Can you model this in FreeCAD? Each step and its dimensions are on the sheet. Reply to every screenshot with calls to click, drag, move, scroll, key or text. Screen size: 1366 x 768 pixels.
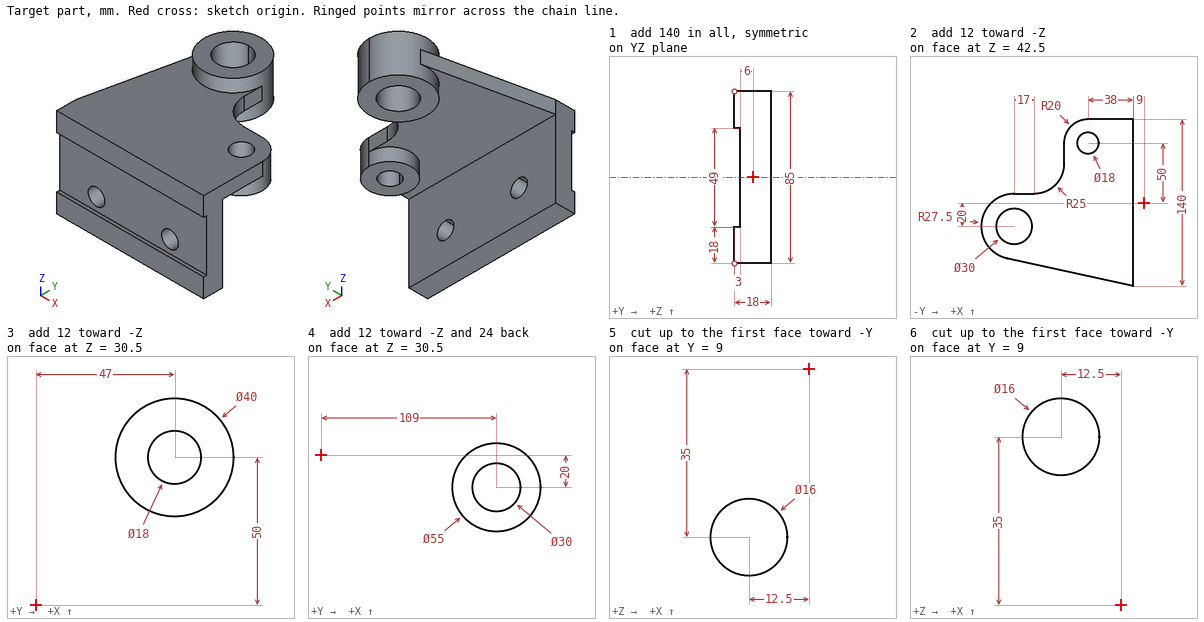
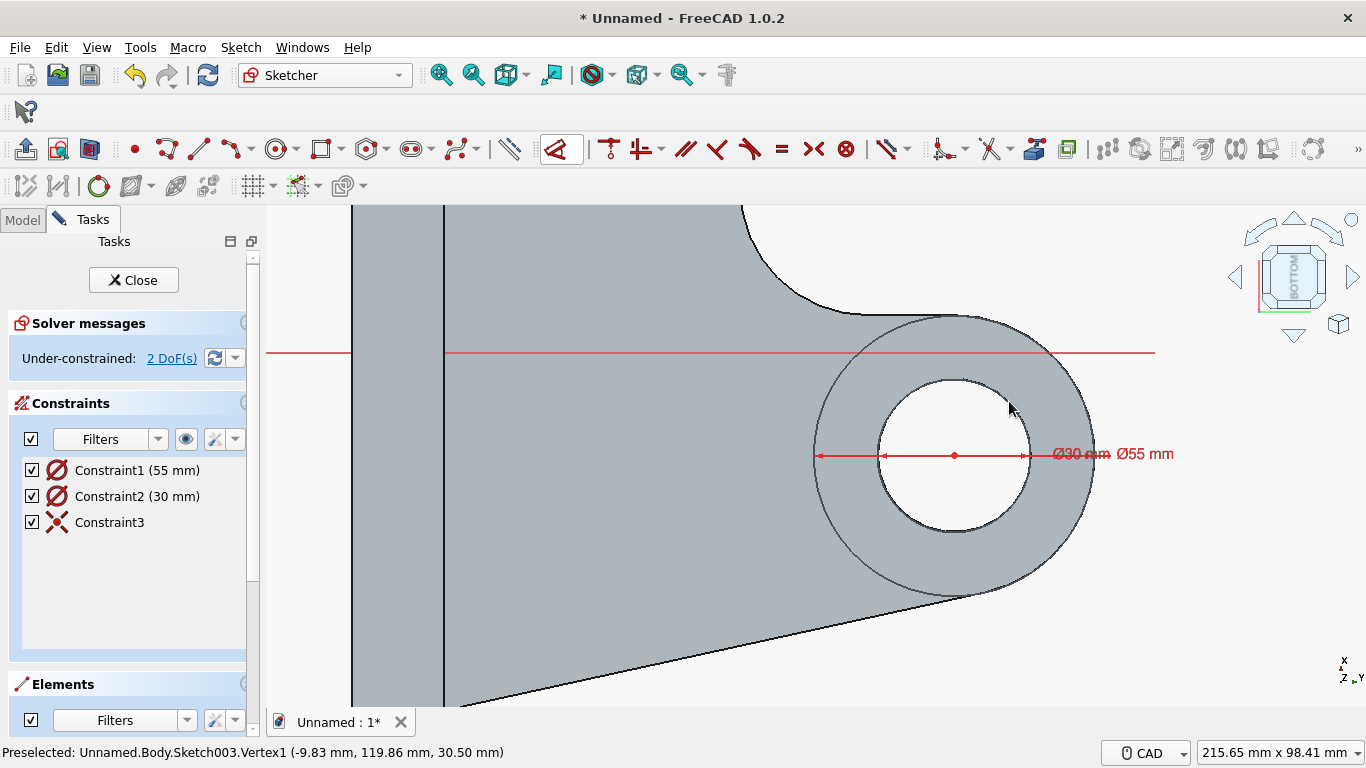
click(954, 456)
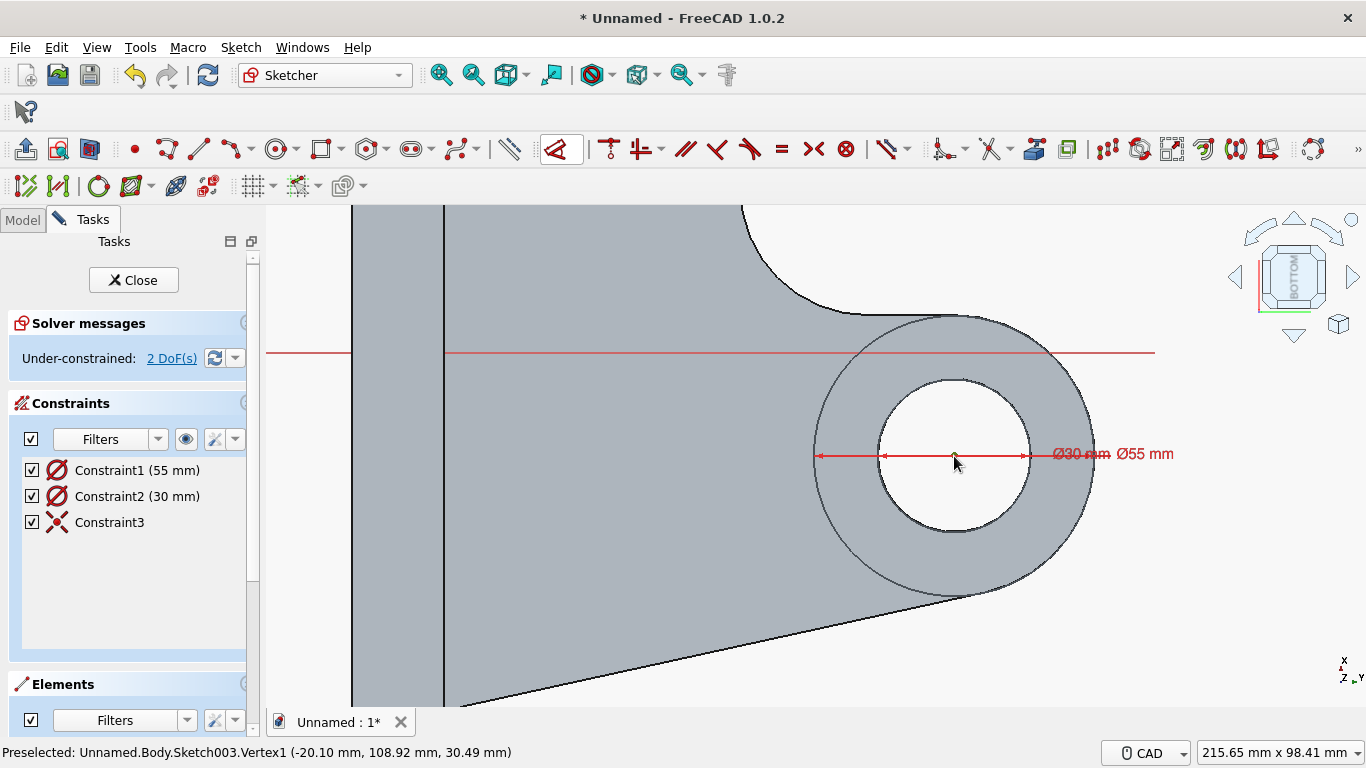
key(i)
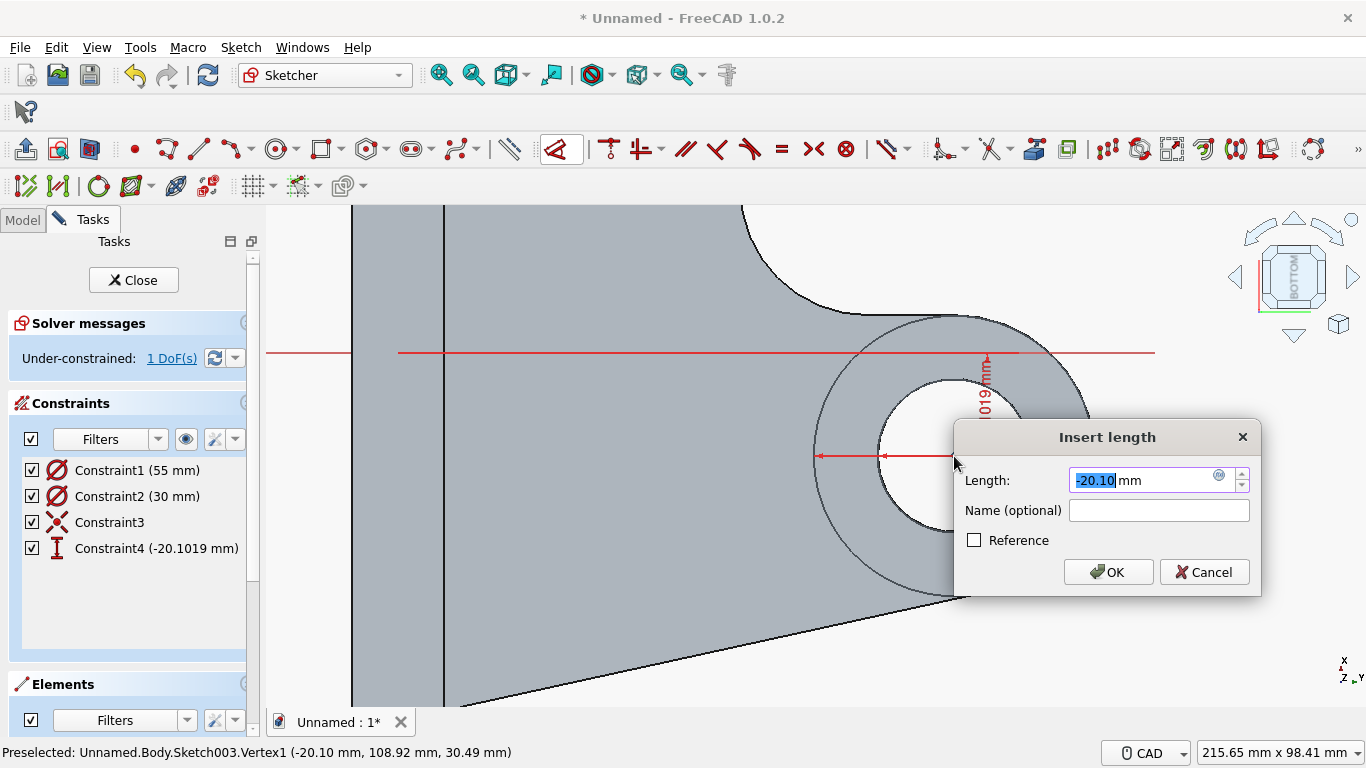
text(-20)
key(Return)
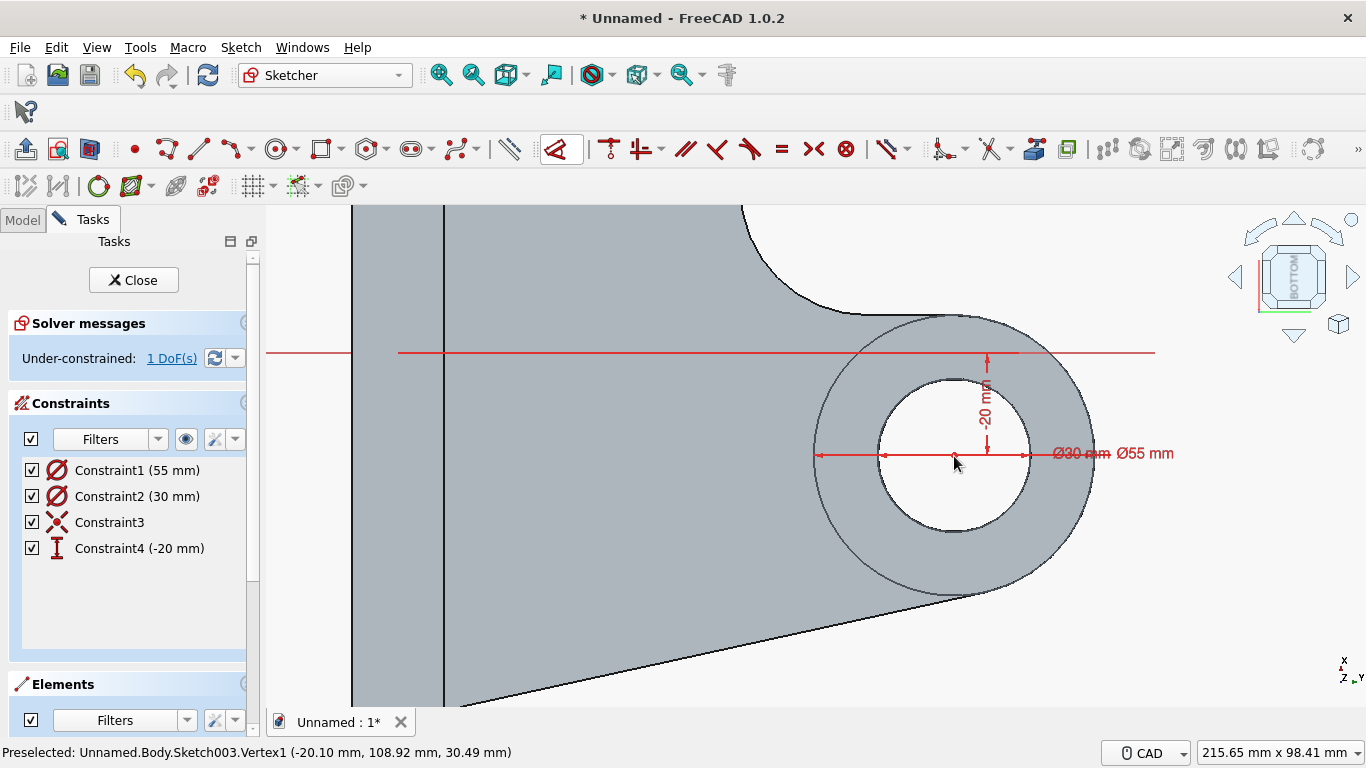
click(954, 455)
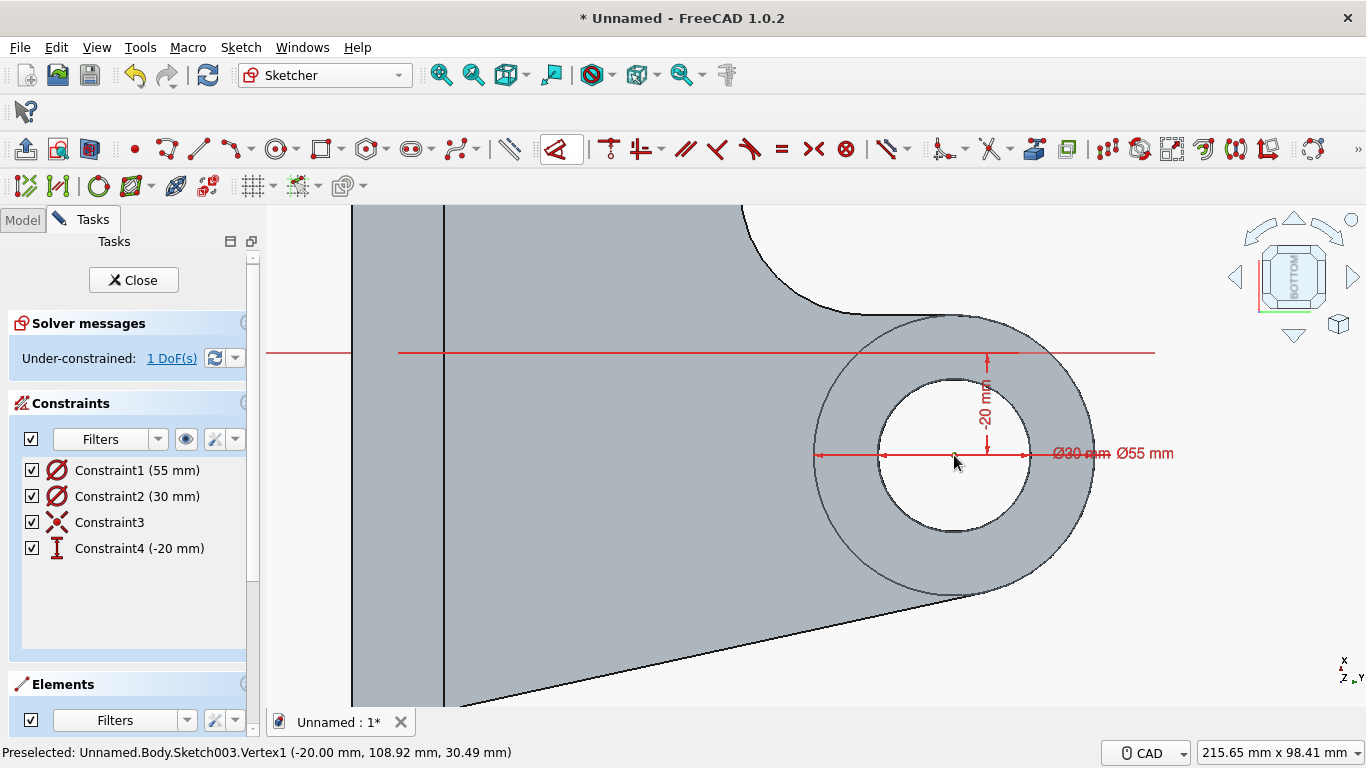
key(l)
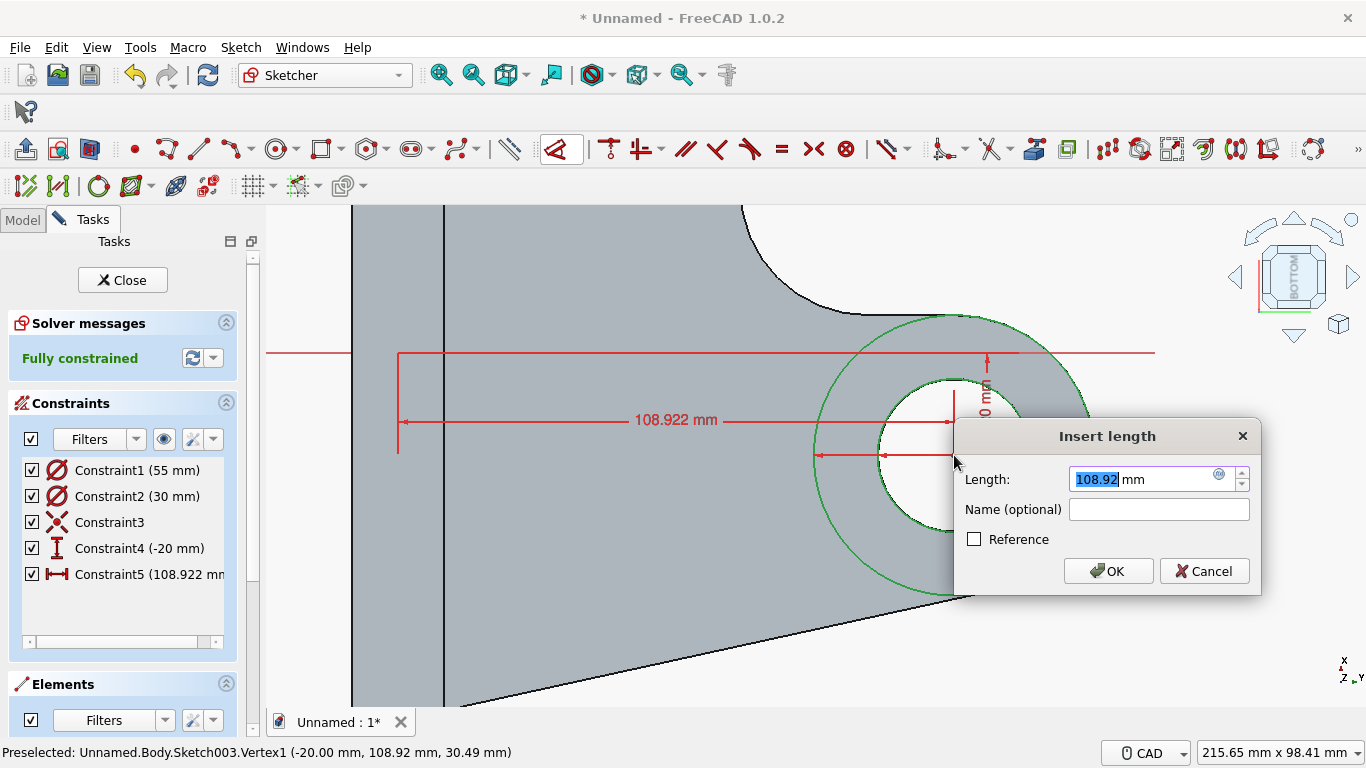
text(109)
key(Return)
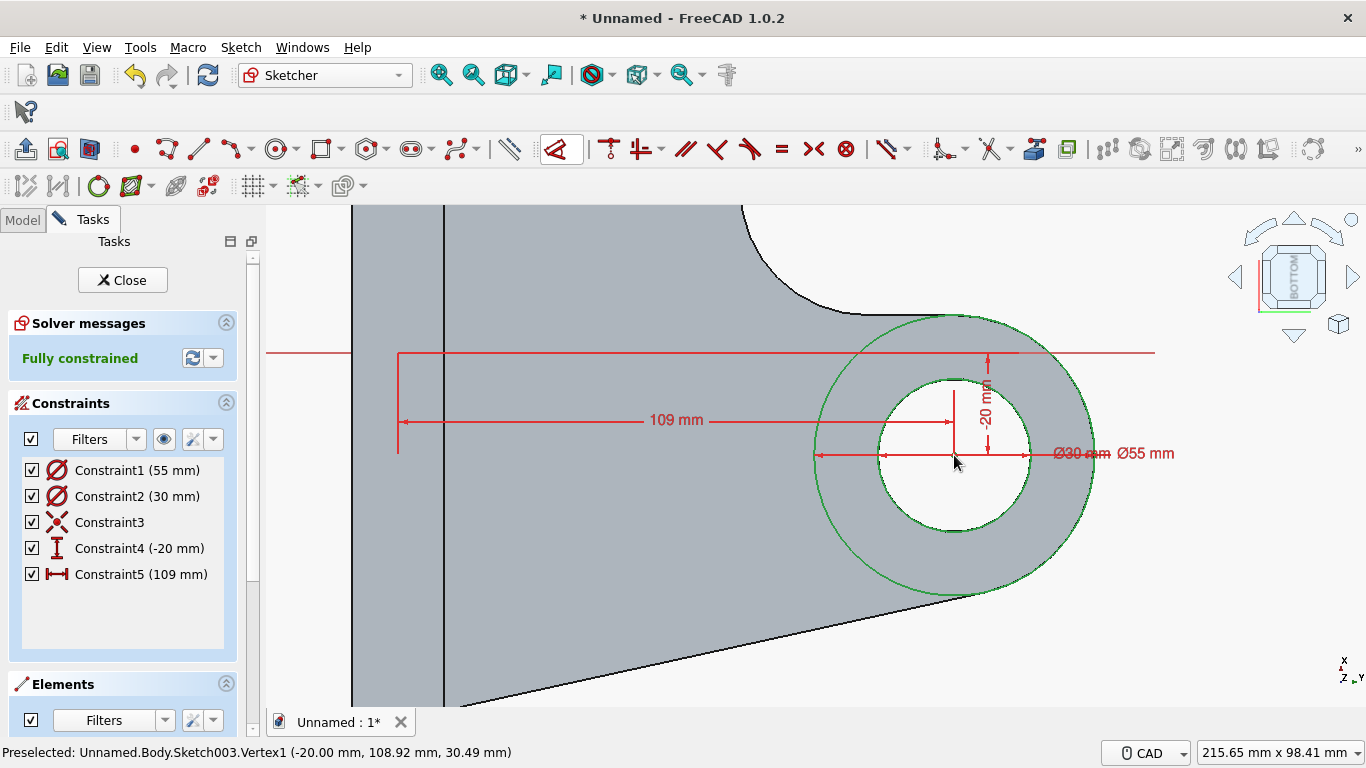
click(123, 280)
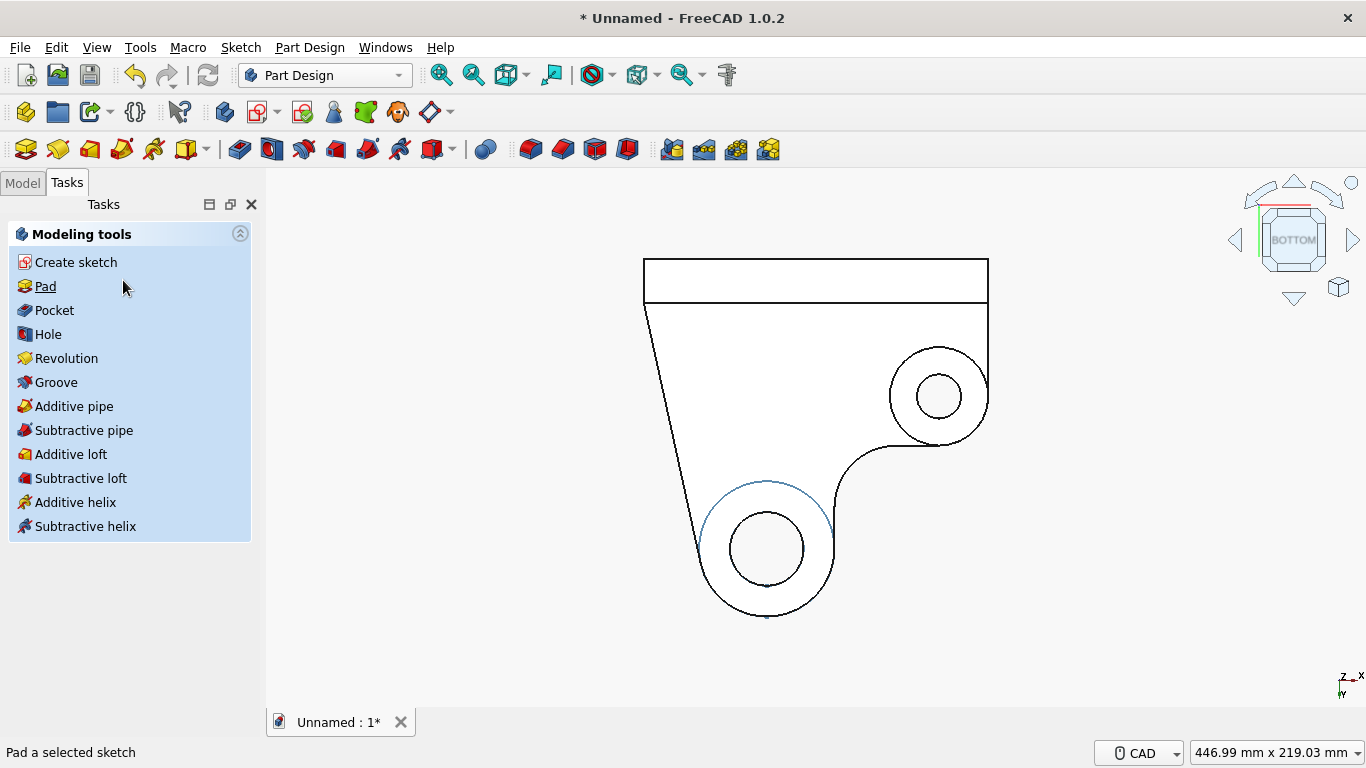
click(26, 150)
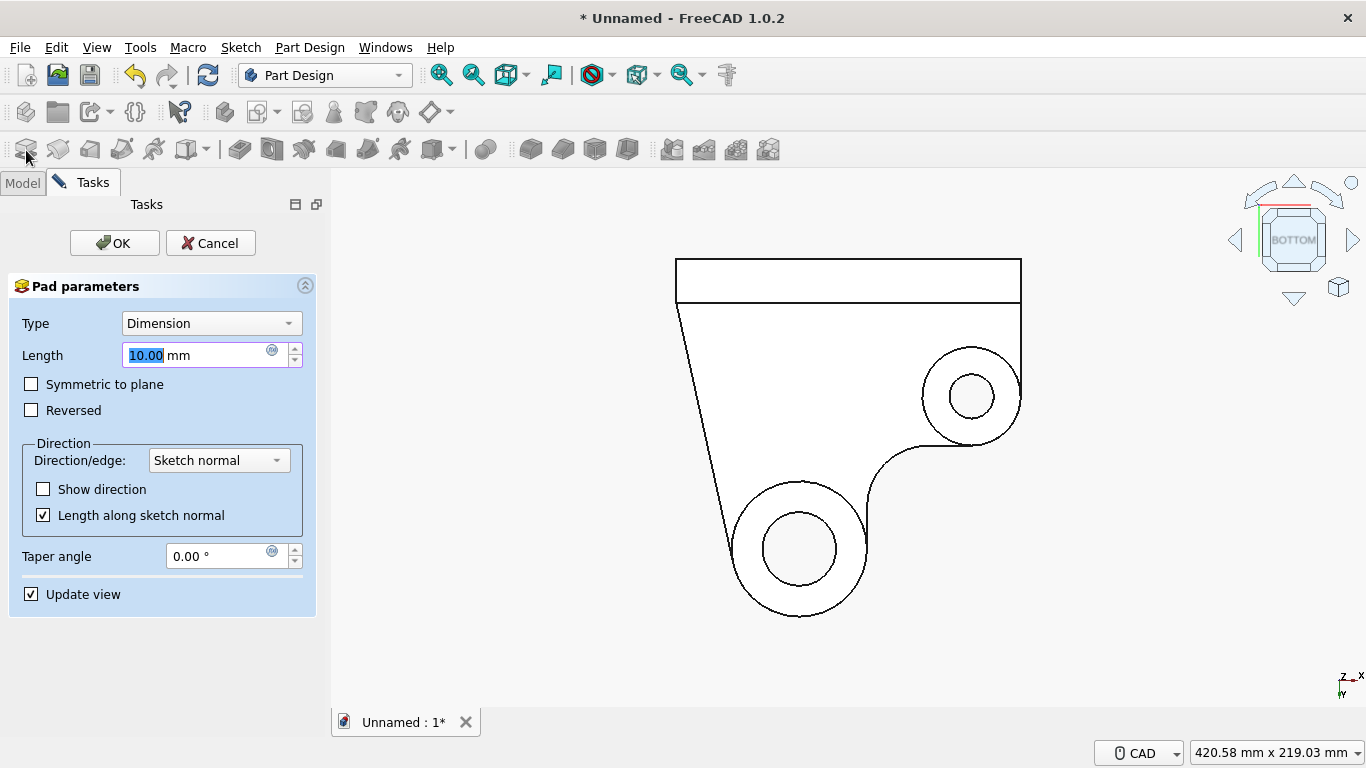
click(212, 324)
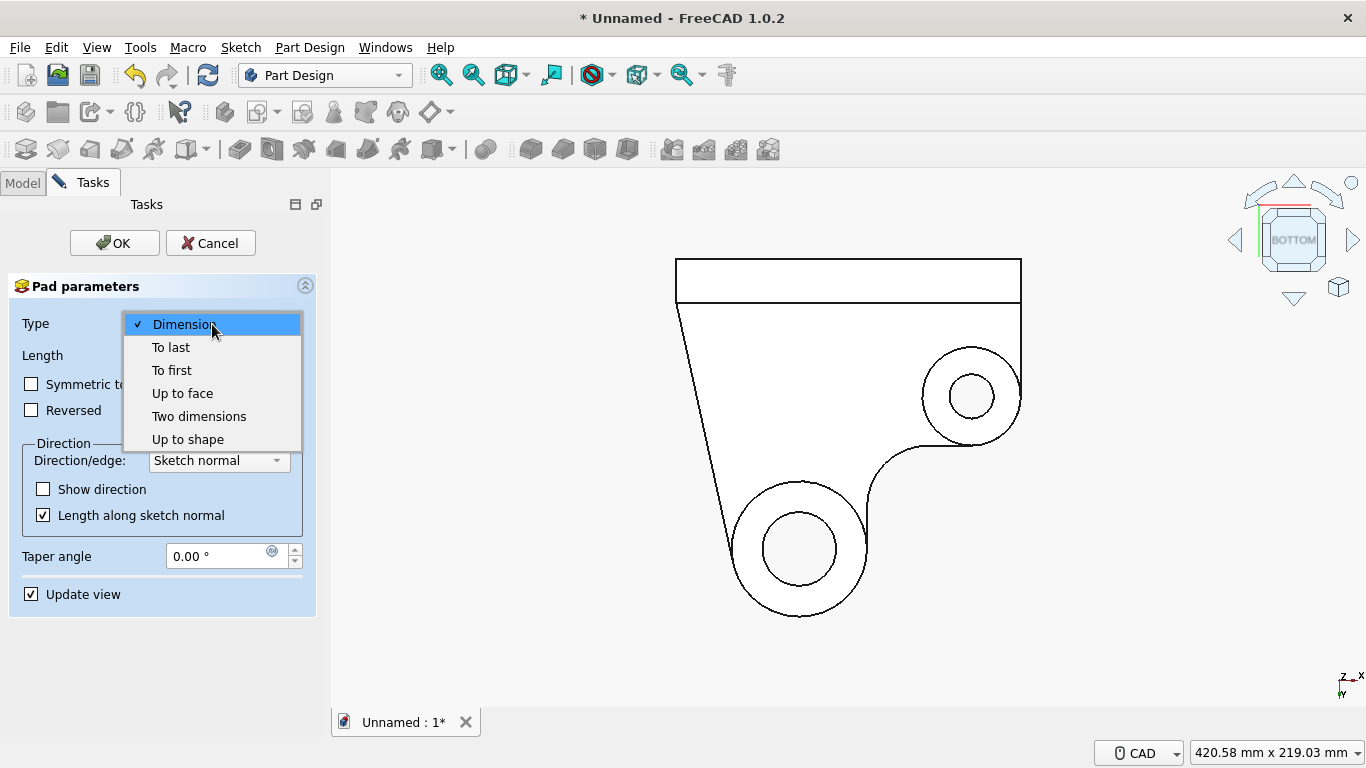
click(212, 416)